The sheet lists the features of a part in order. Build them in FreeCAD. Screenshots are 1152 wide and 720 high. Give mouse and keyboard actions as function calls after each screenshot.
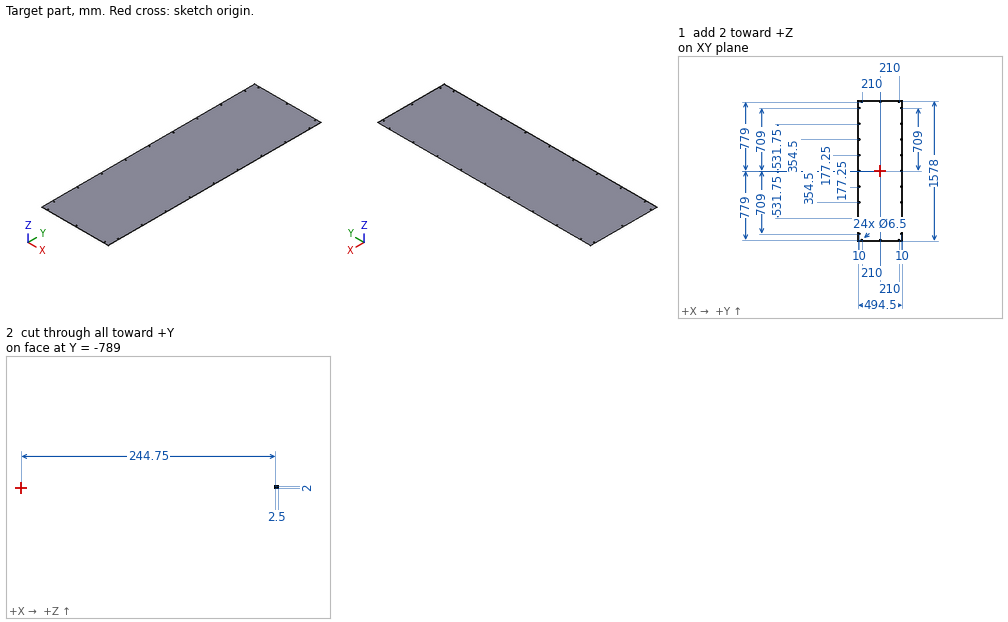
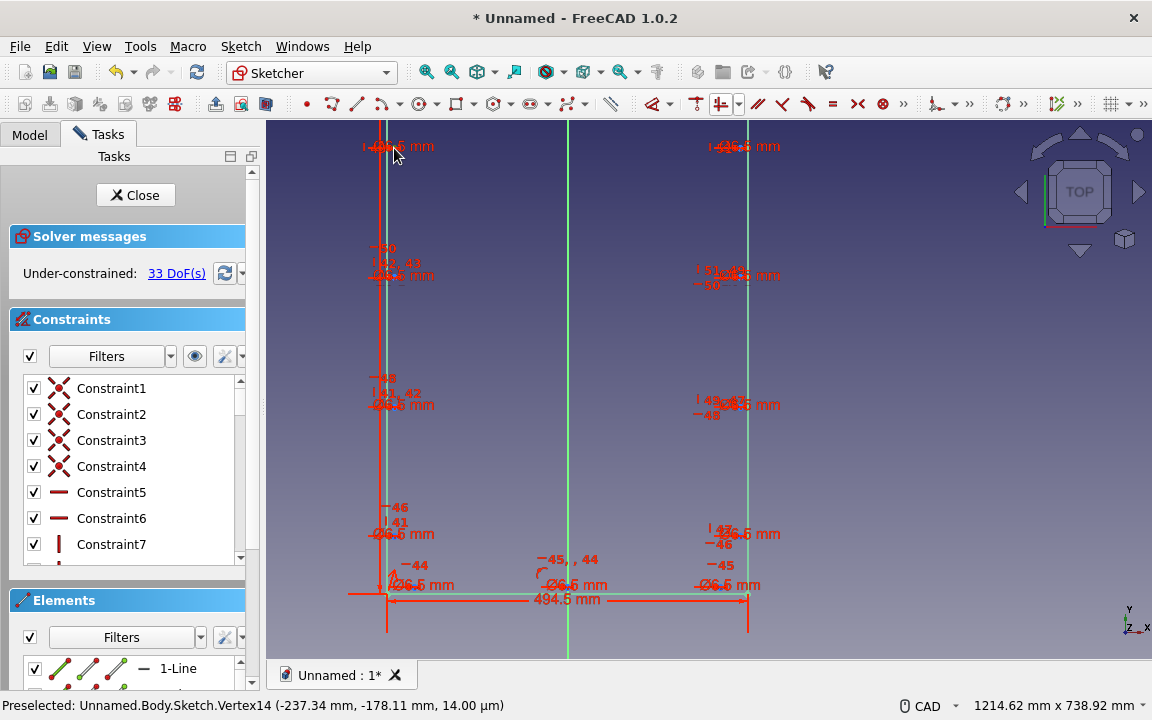
click(741, 148)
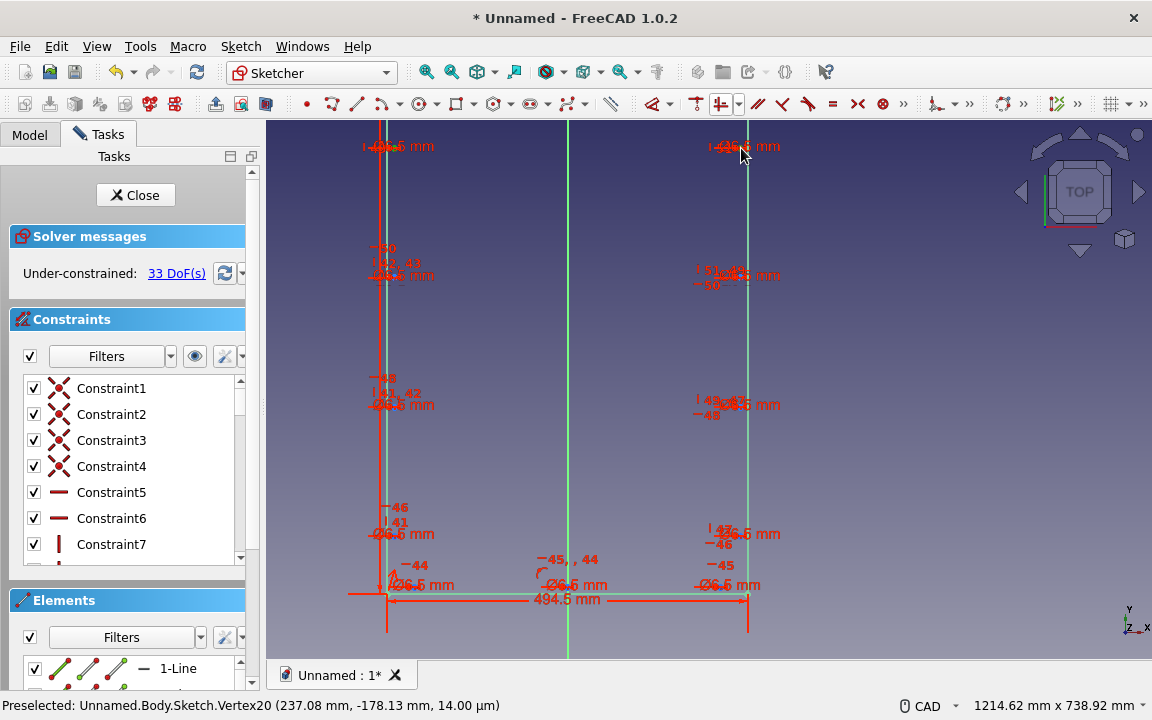
key(h)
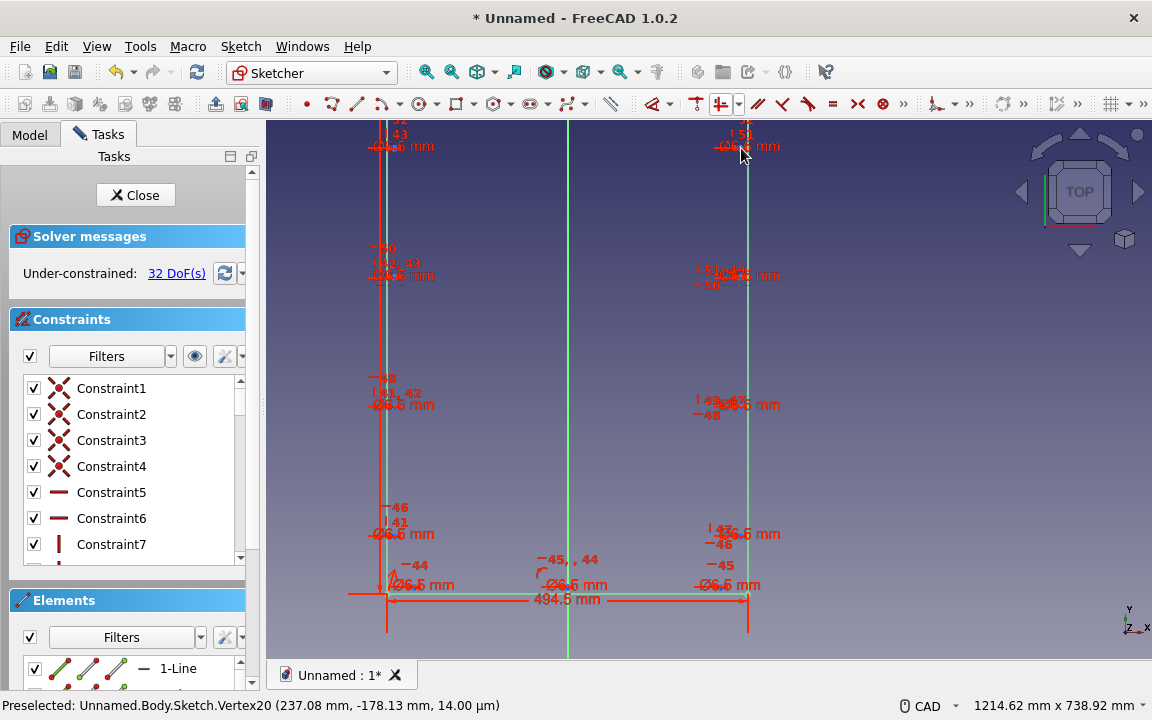
click(394, 148)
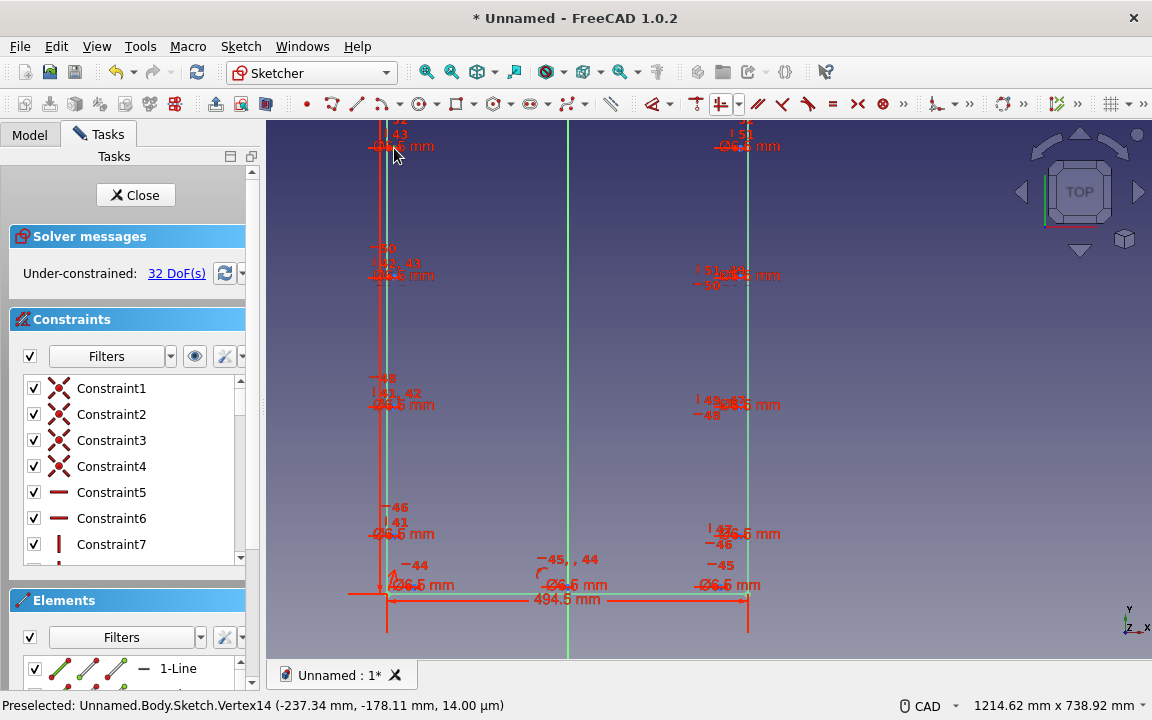
scroll(672, 549, down, 6)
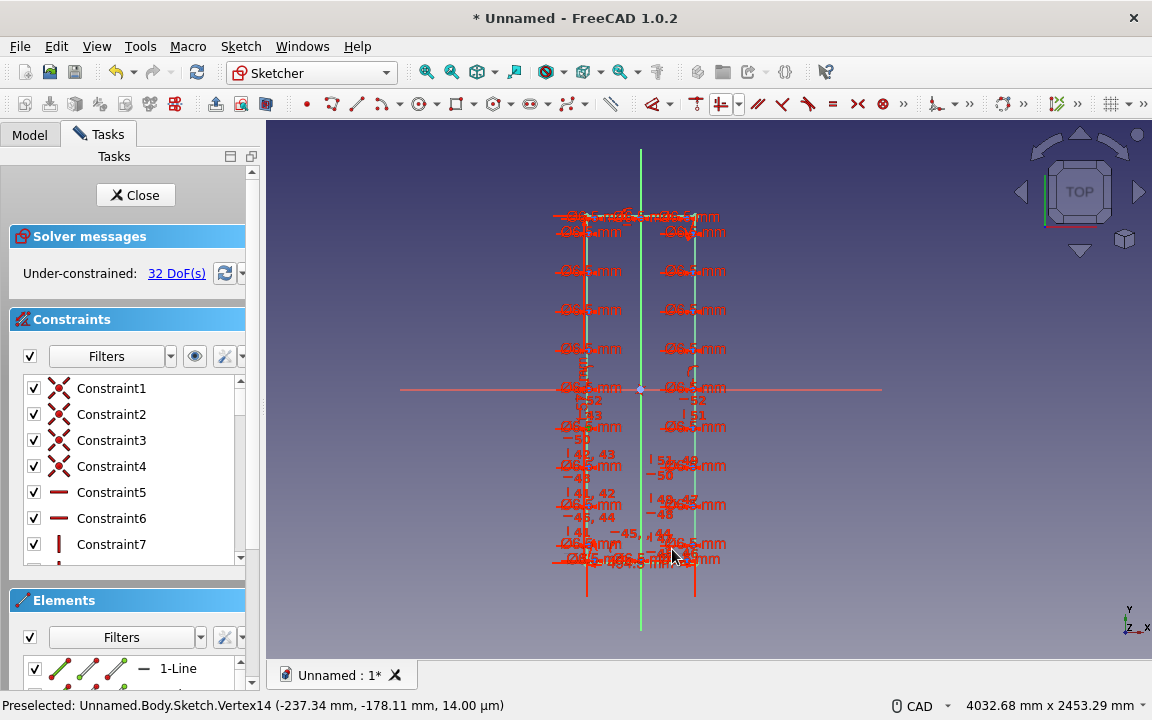
click(589, 390)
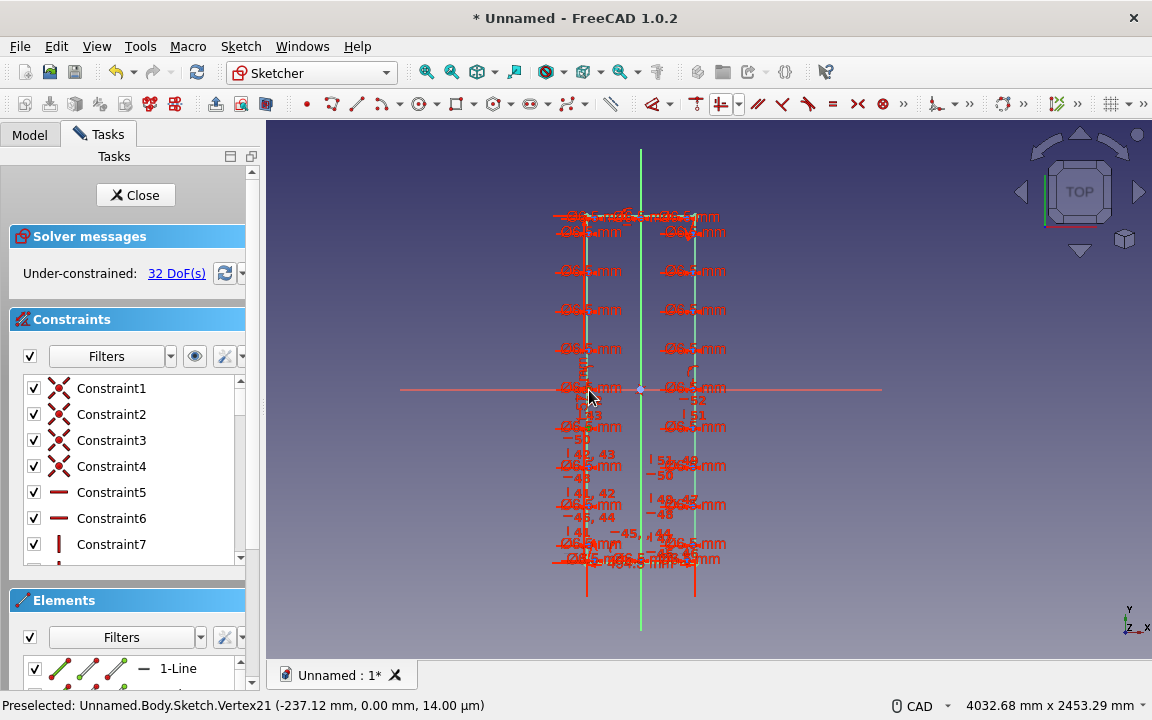
key(v)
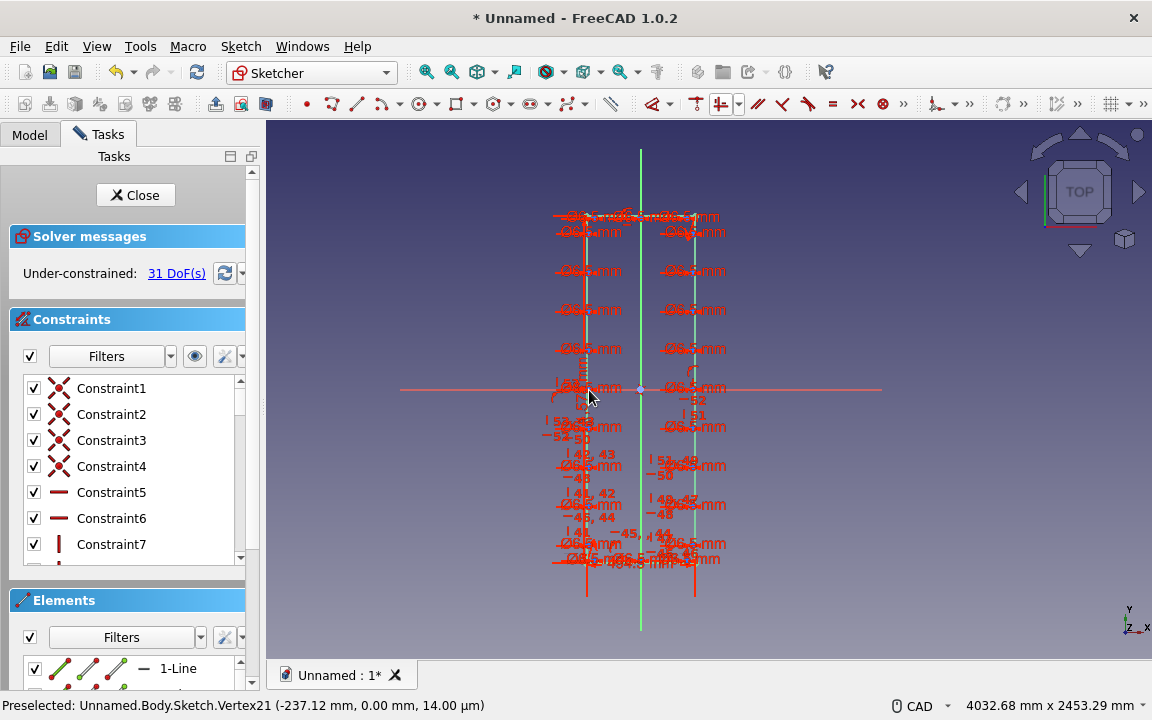
click(589, 390)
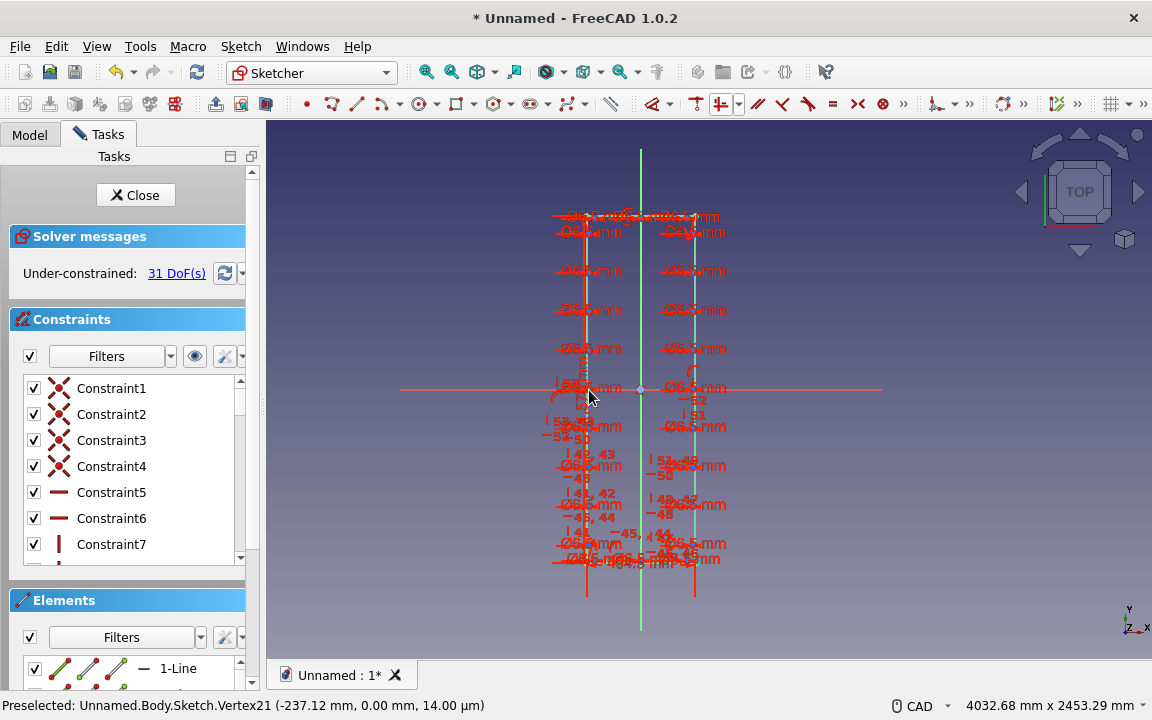
click(589, 351)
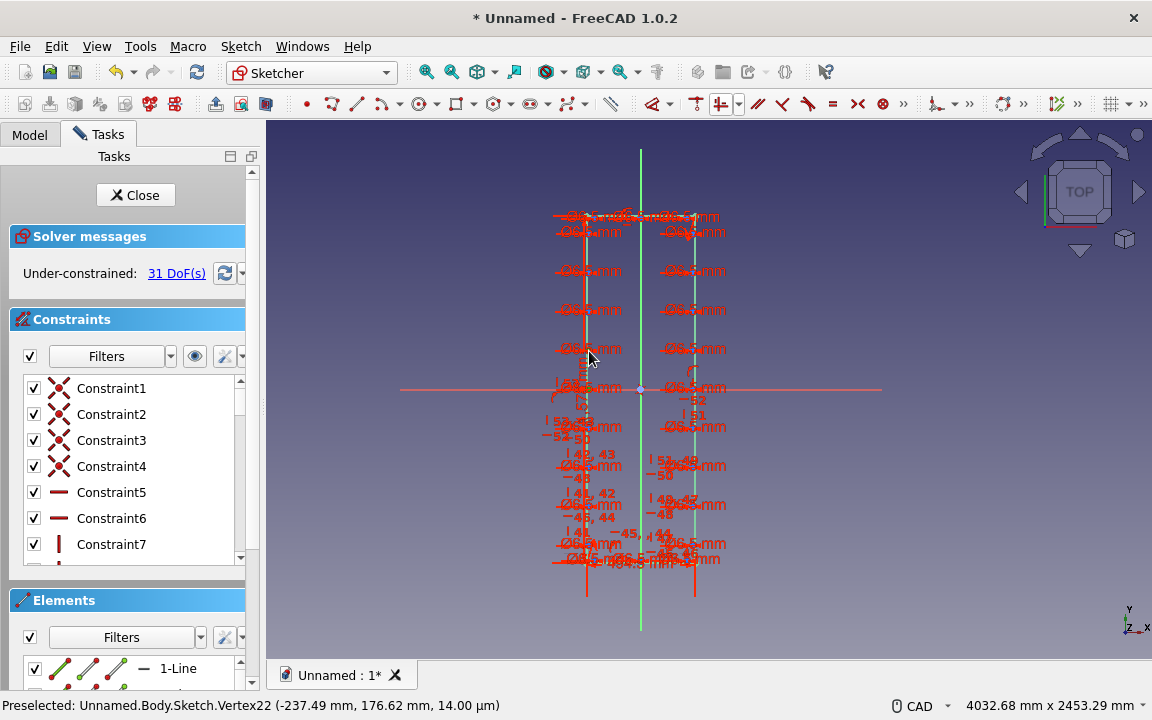
key(v)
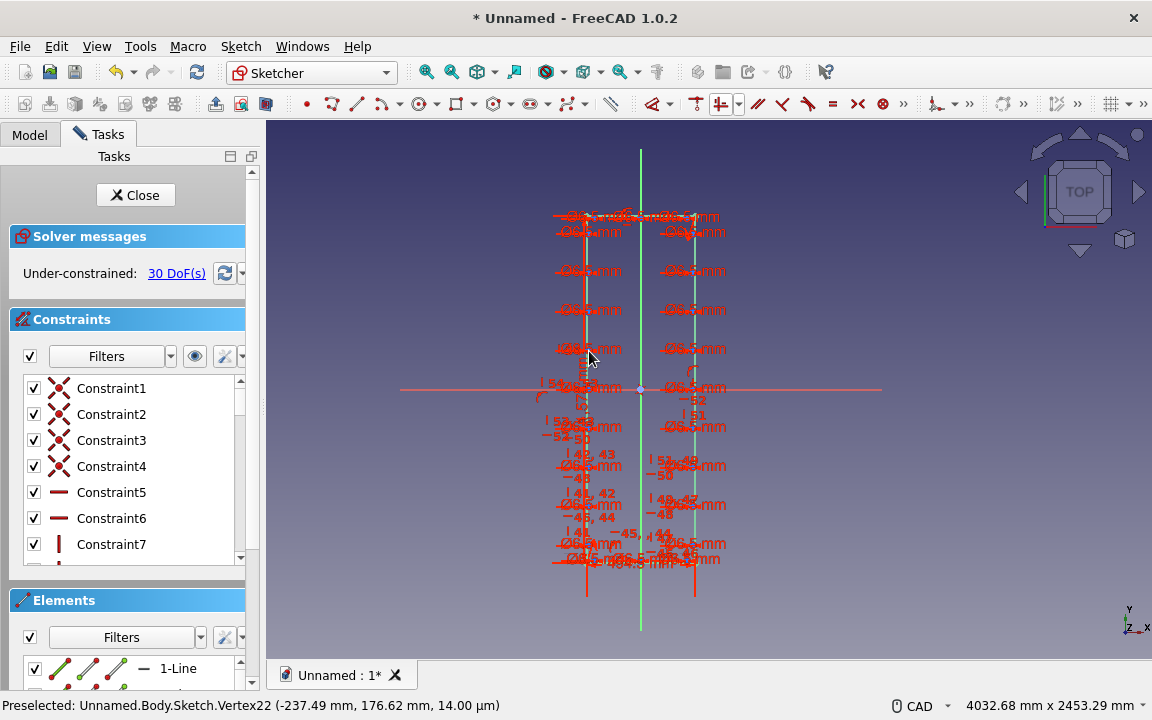
click(589, 351)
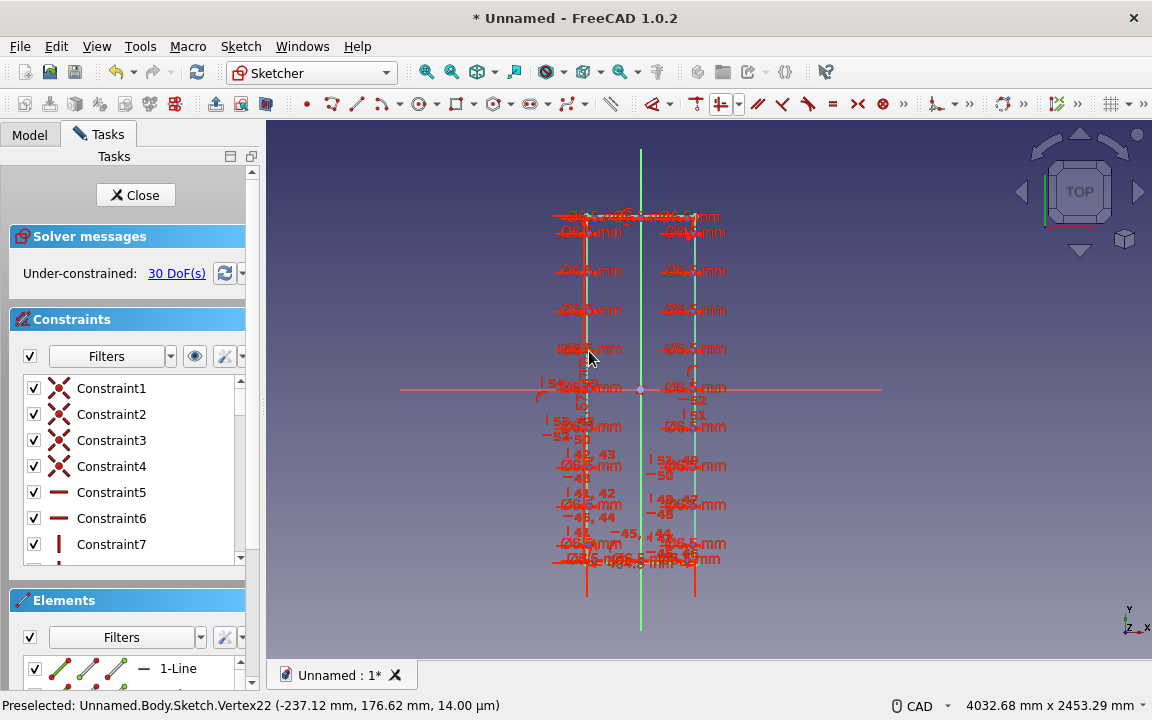
click(589, 312)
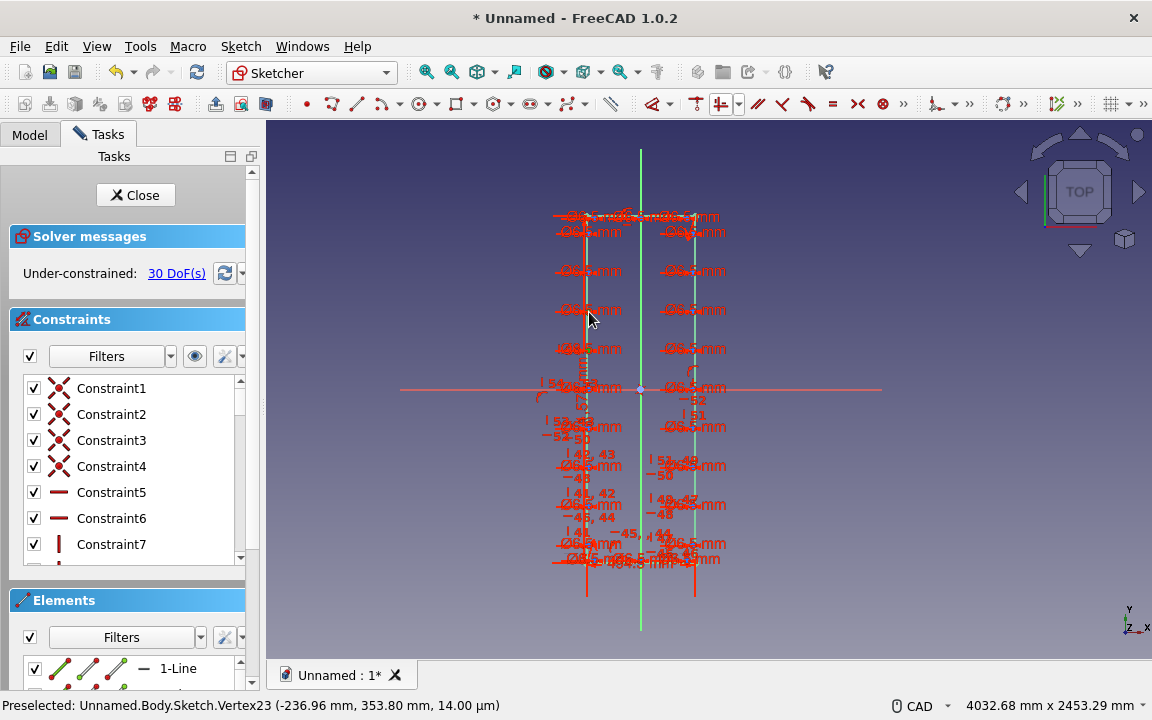
key(v)